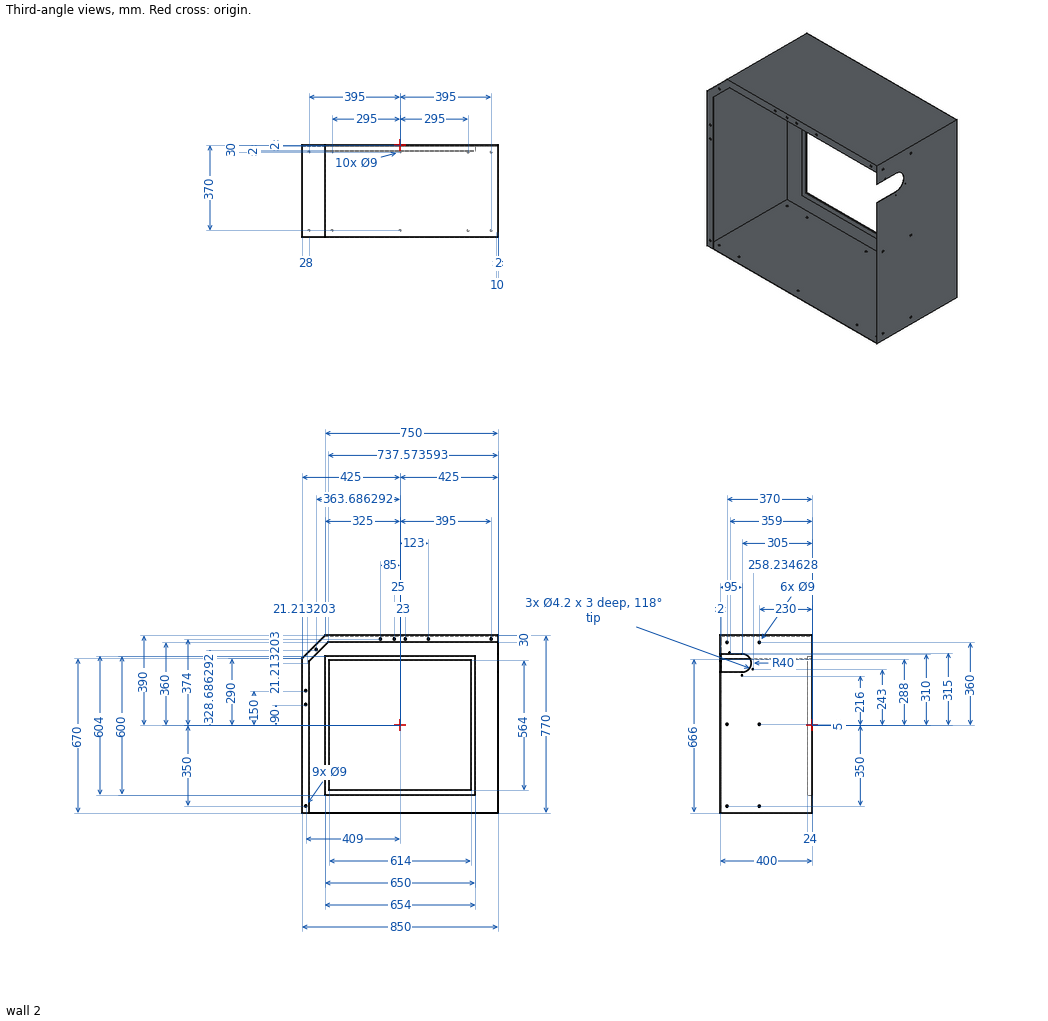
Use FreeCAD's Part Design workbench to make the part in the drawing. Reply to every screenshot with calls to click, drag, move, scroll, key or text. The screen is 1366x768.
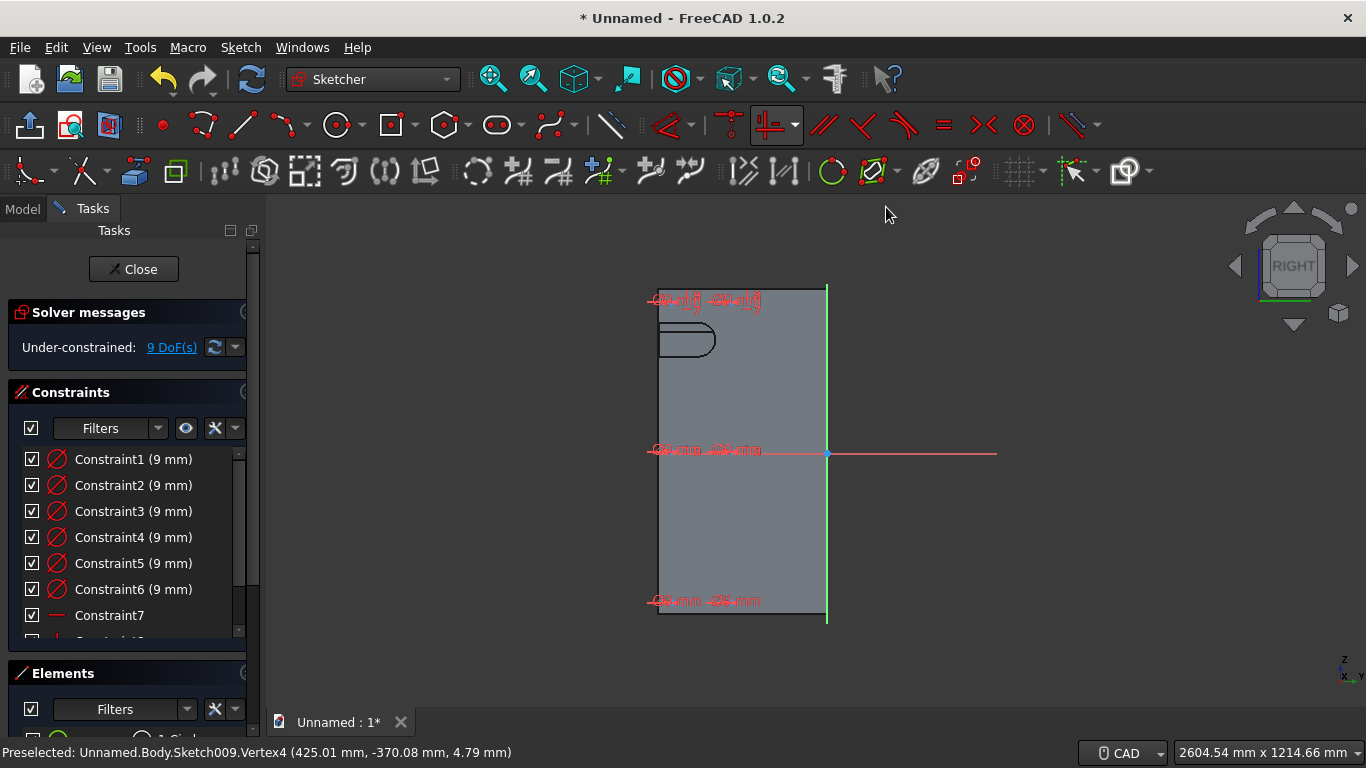
click(731, 452)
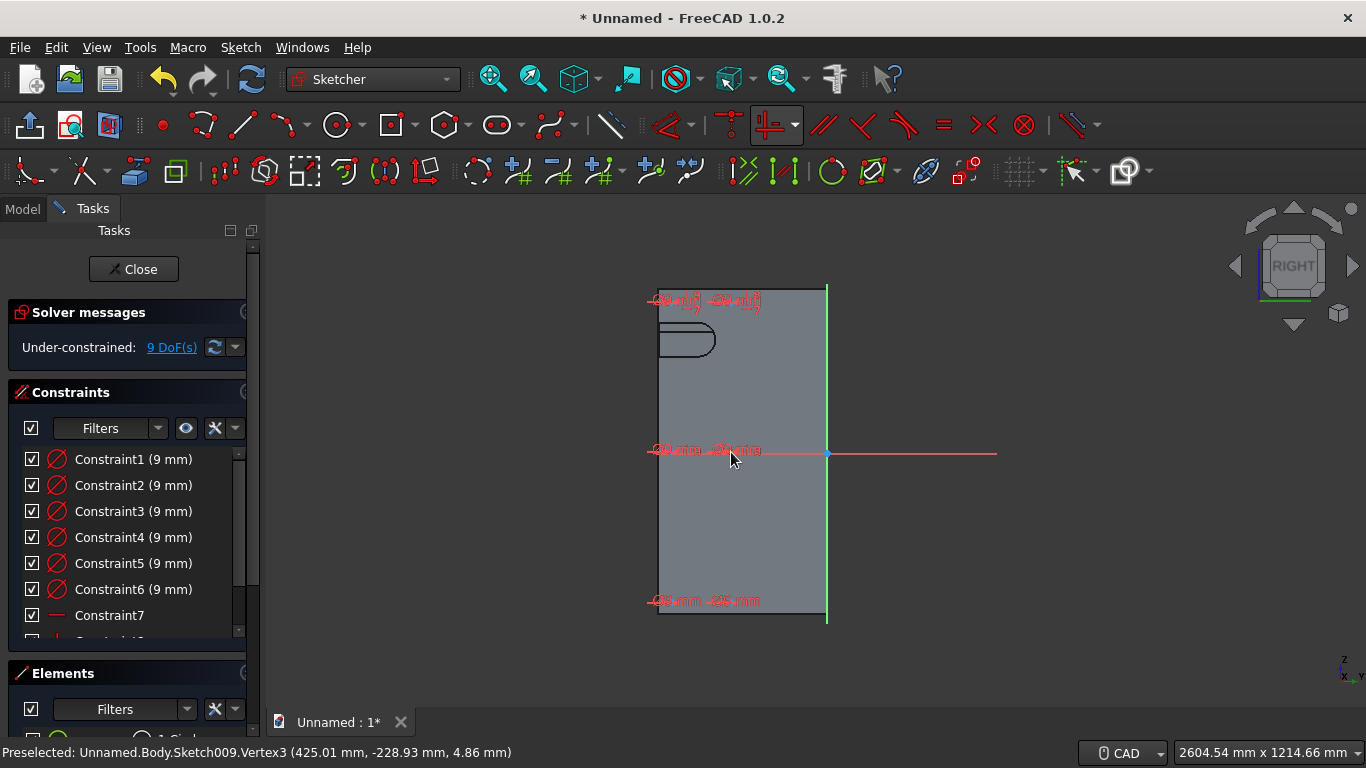
click(671, 452)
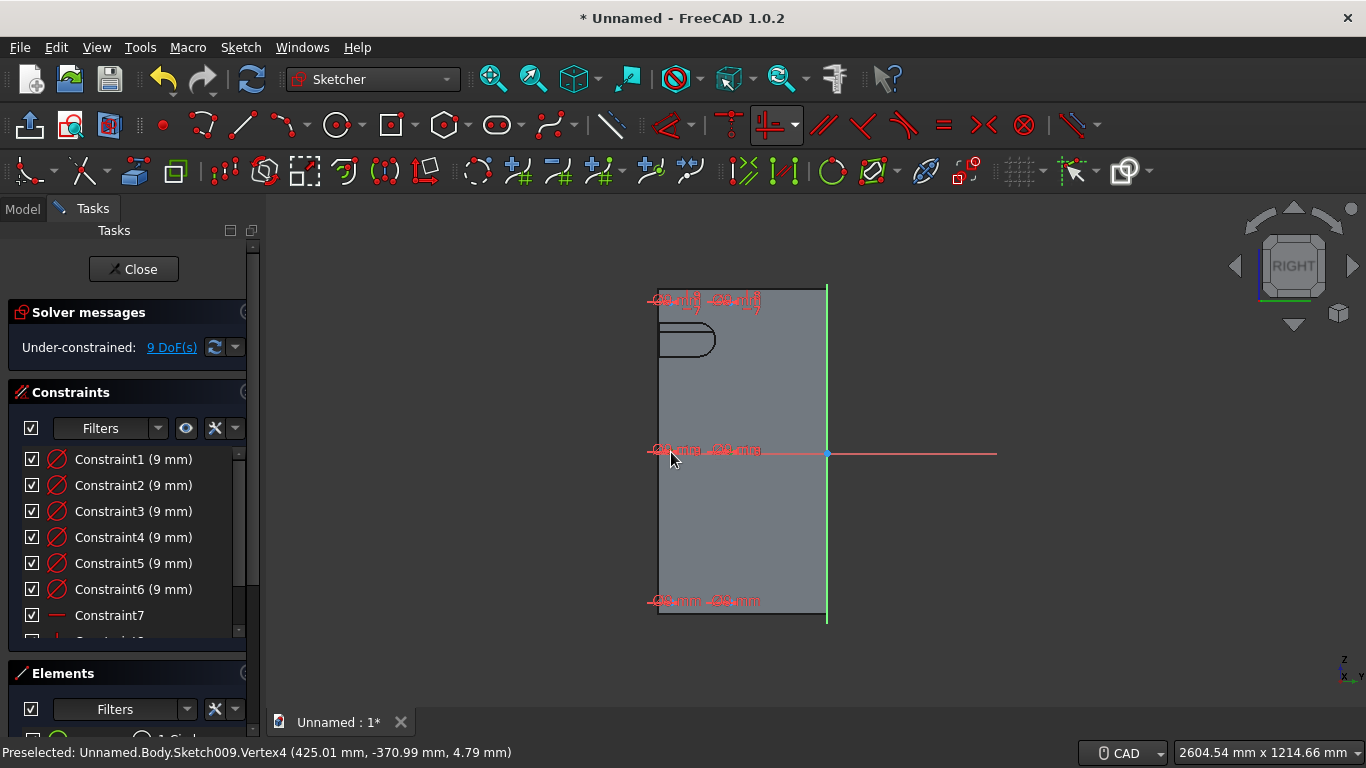
click(798, 126)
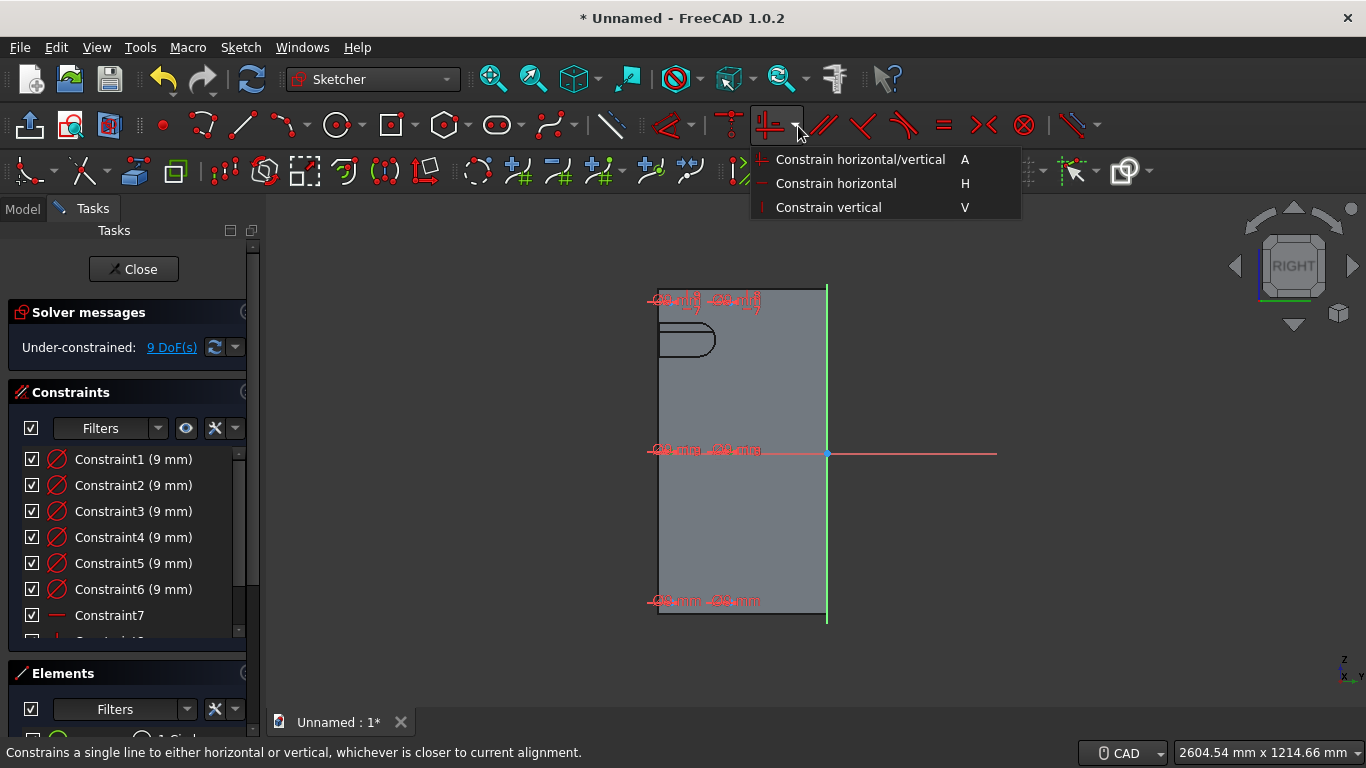
click(886, 183)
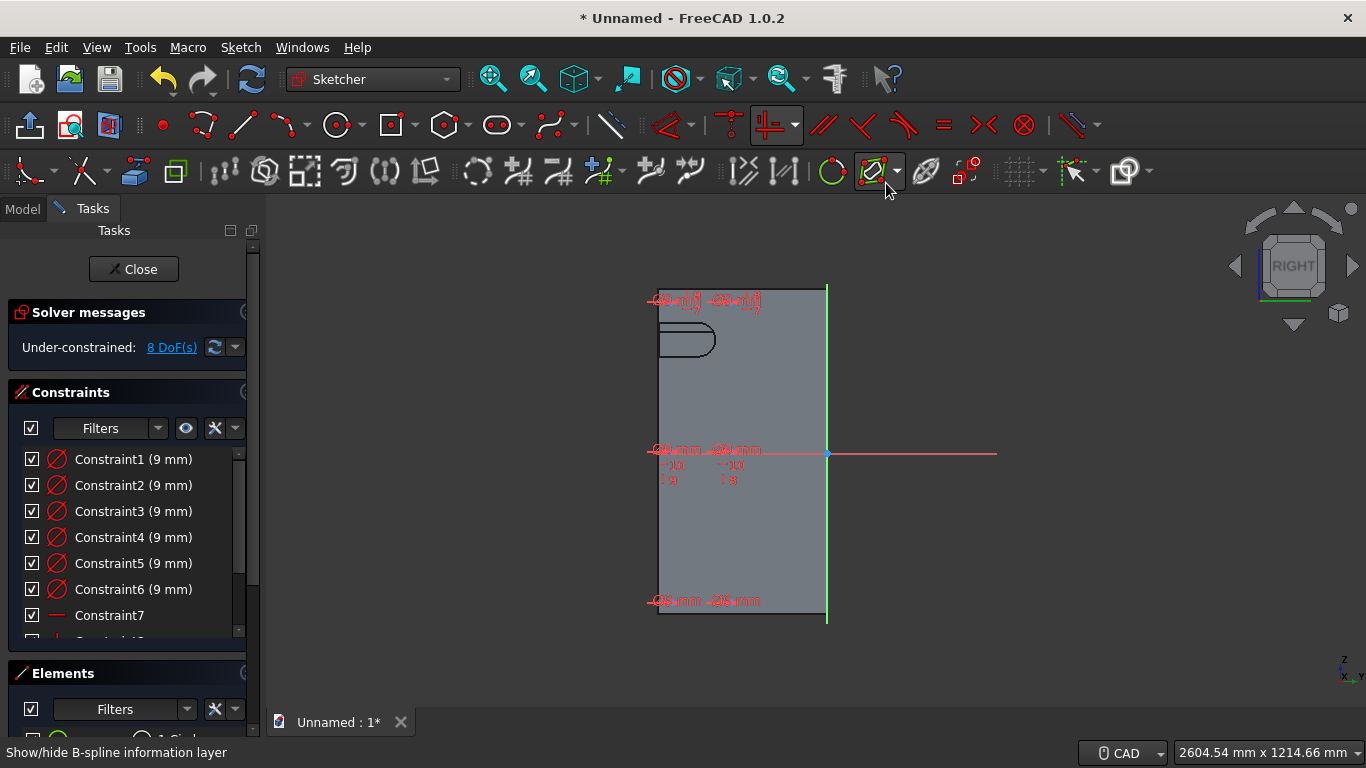
click(671, 452)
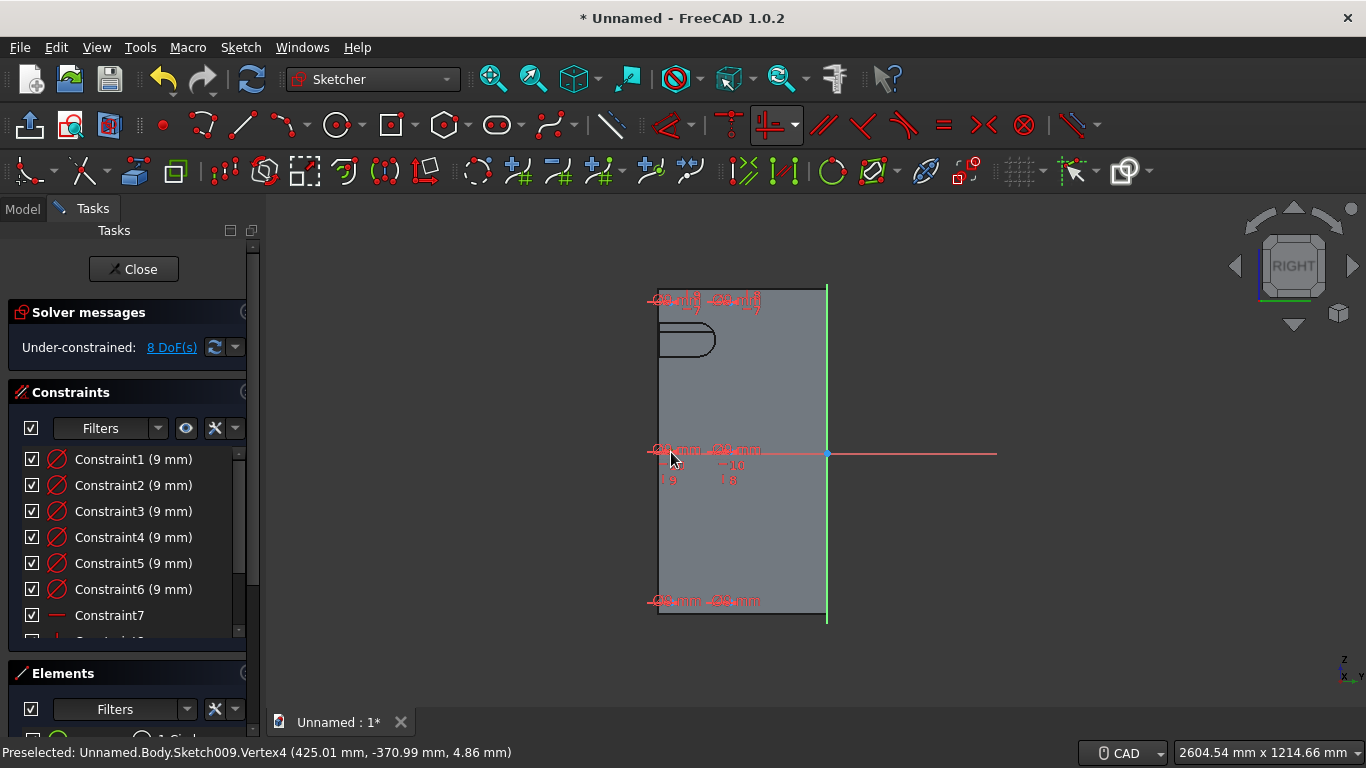
click(671, 603)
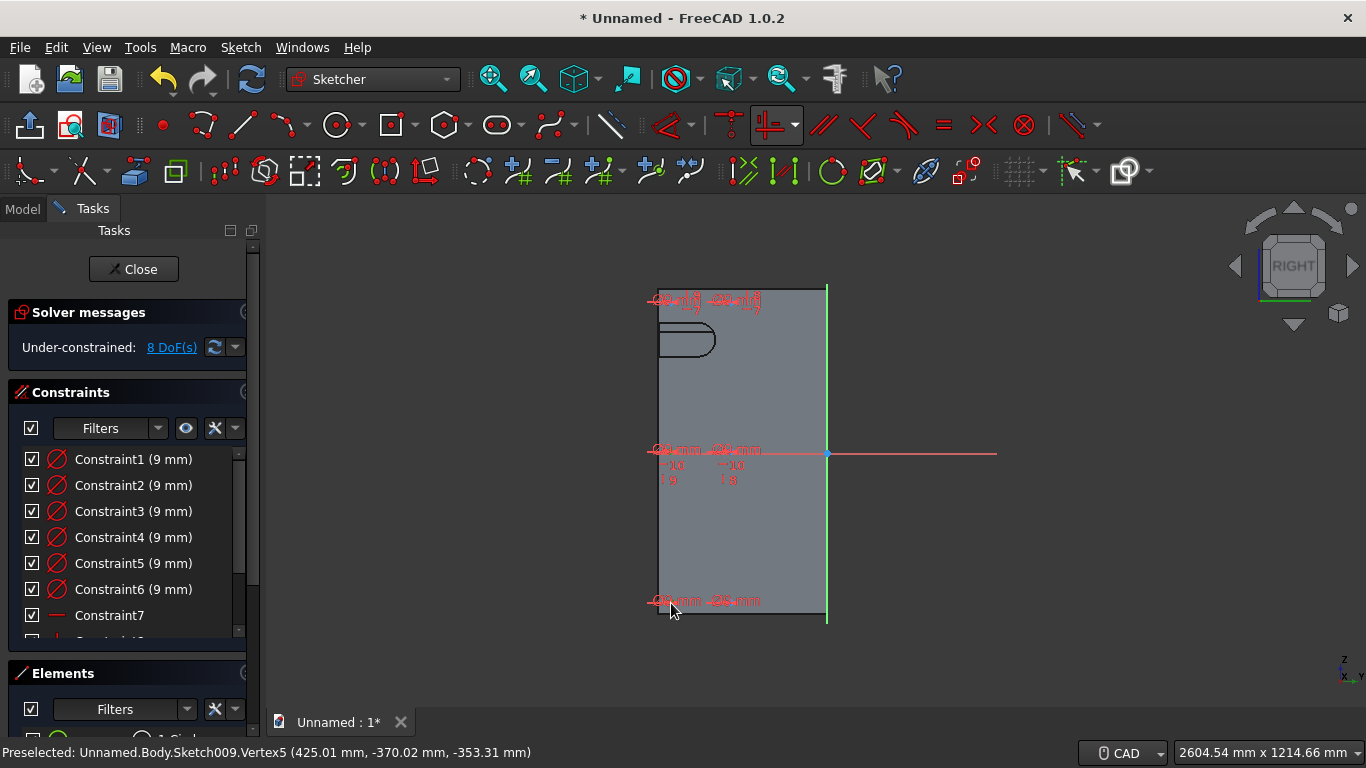
click(798, 126)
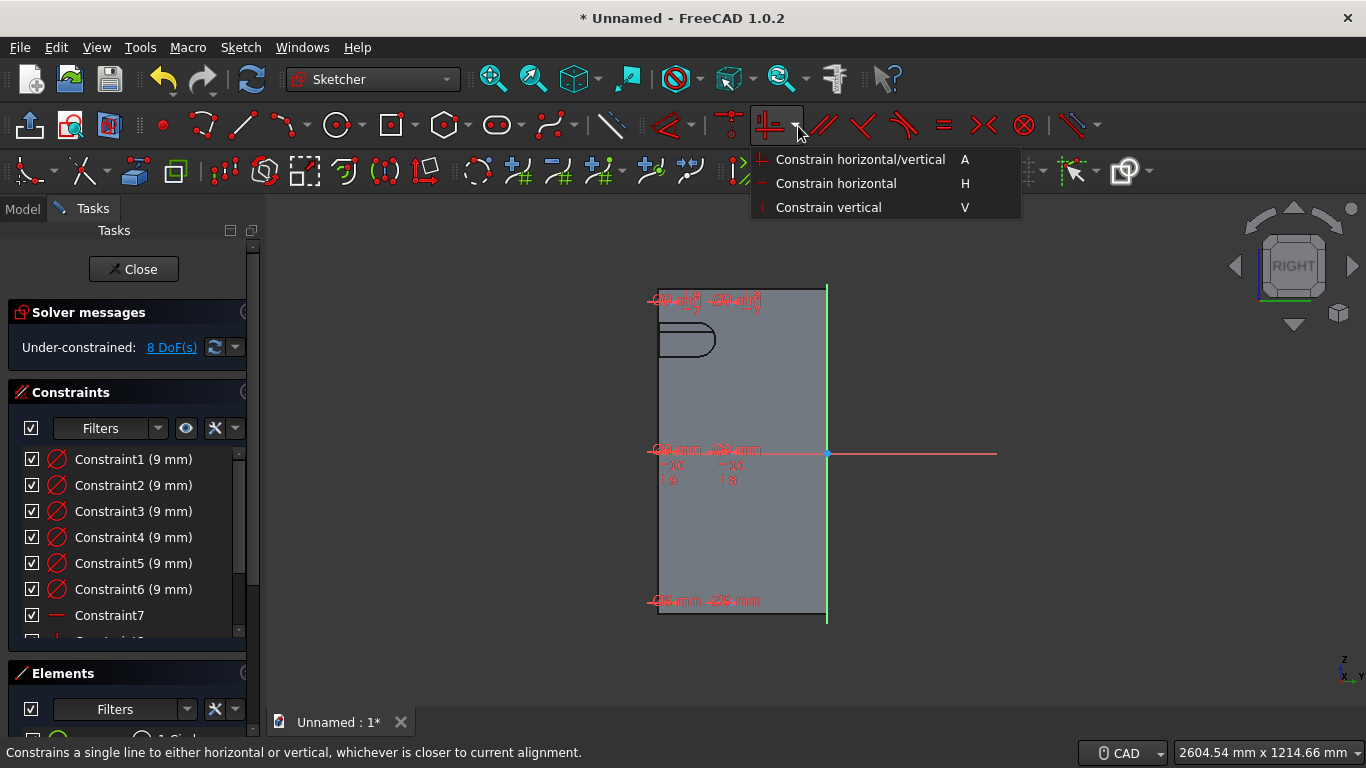
click(886, 207)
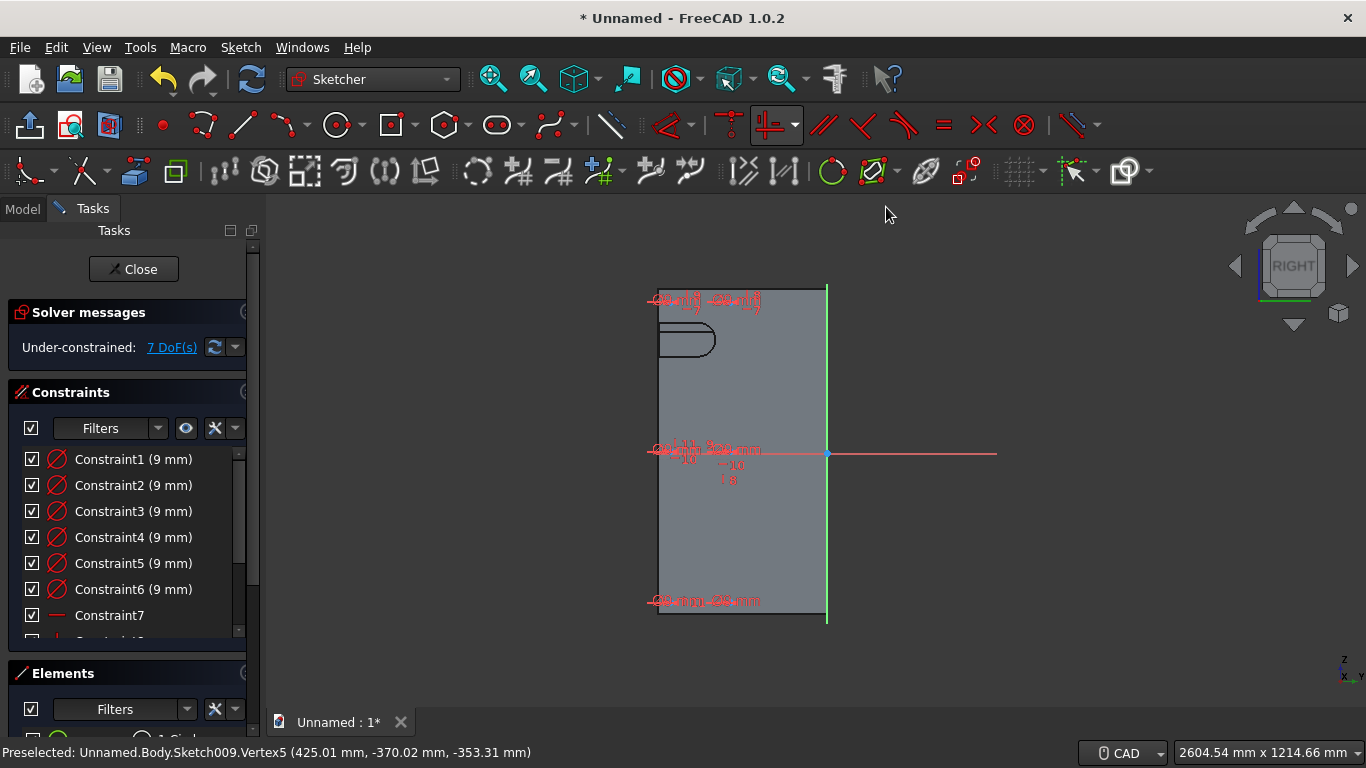
click(731, 452)